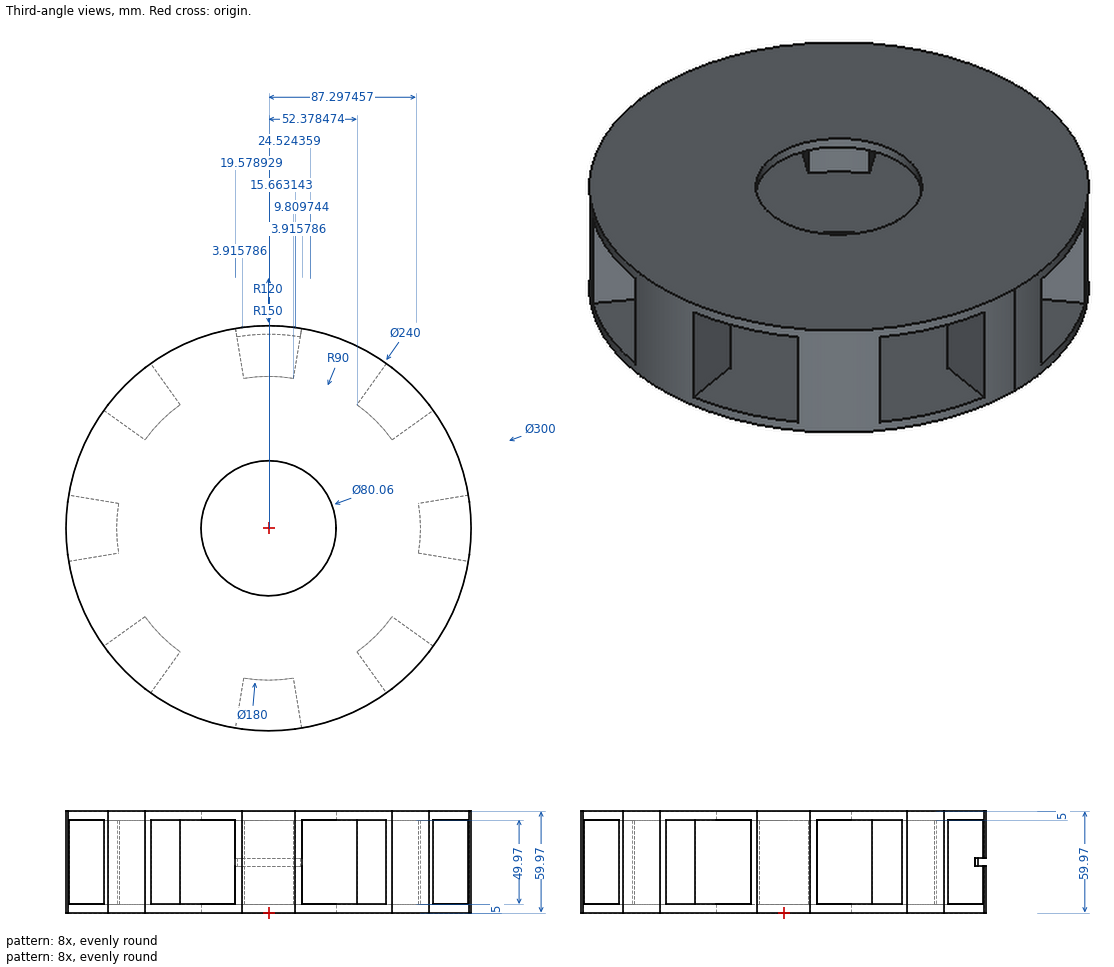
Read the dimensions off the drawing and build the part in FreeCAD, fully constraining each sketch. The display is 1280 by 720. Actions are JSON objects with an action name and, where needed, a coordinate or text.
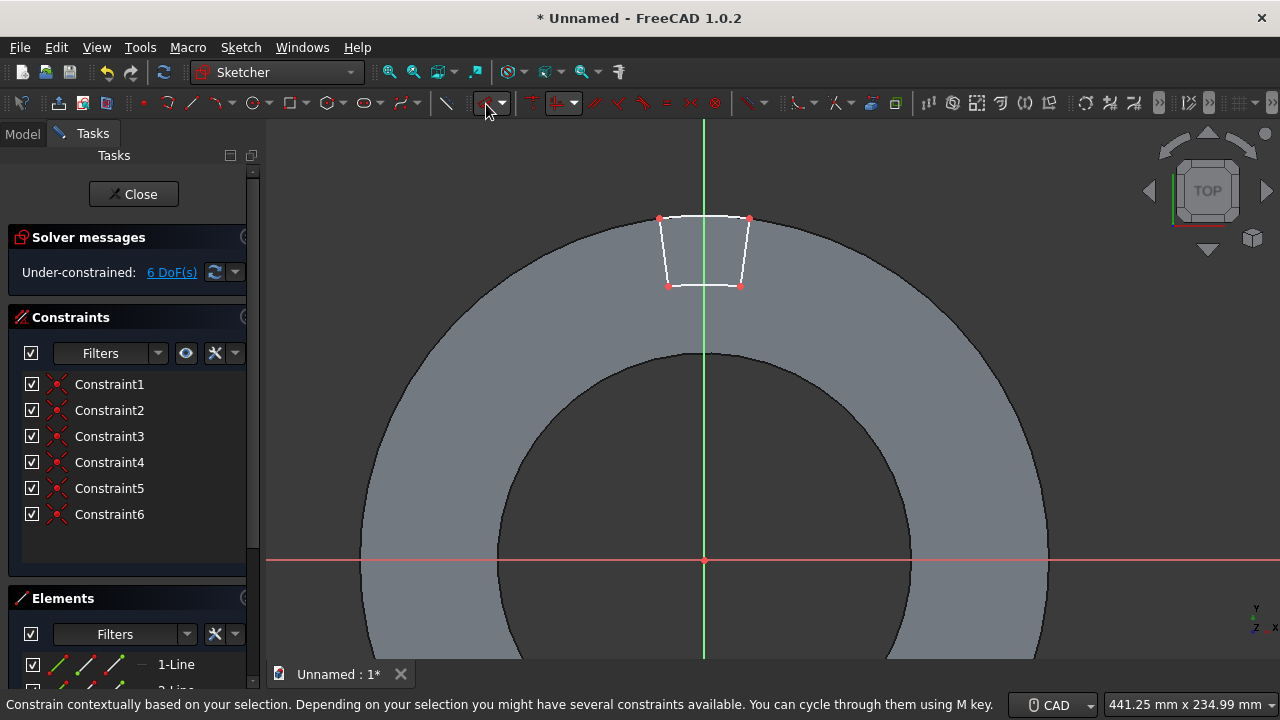
{"action": "left_click", "coordinate": [719, 285]}
{"action": "left_click", "coordinate": [721, 253]}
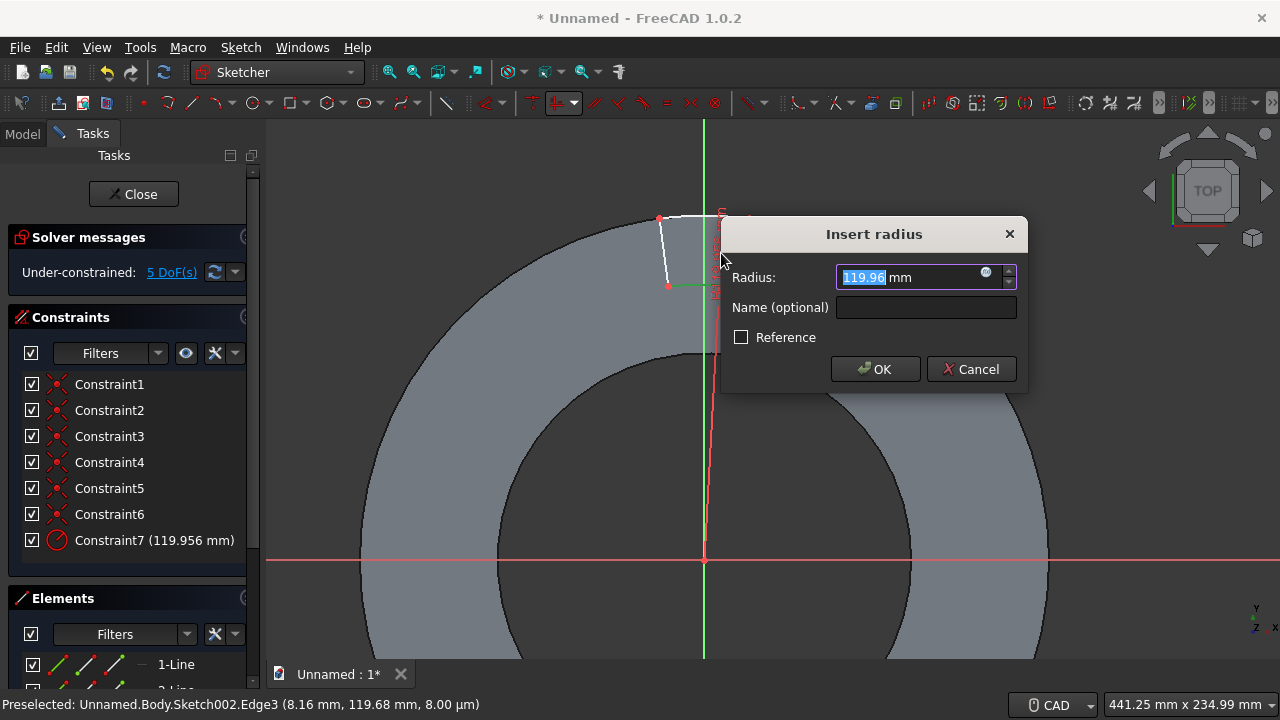
{"action": "type", "text": "120"}
{"action": "key", "text": "Return"}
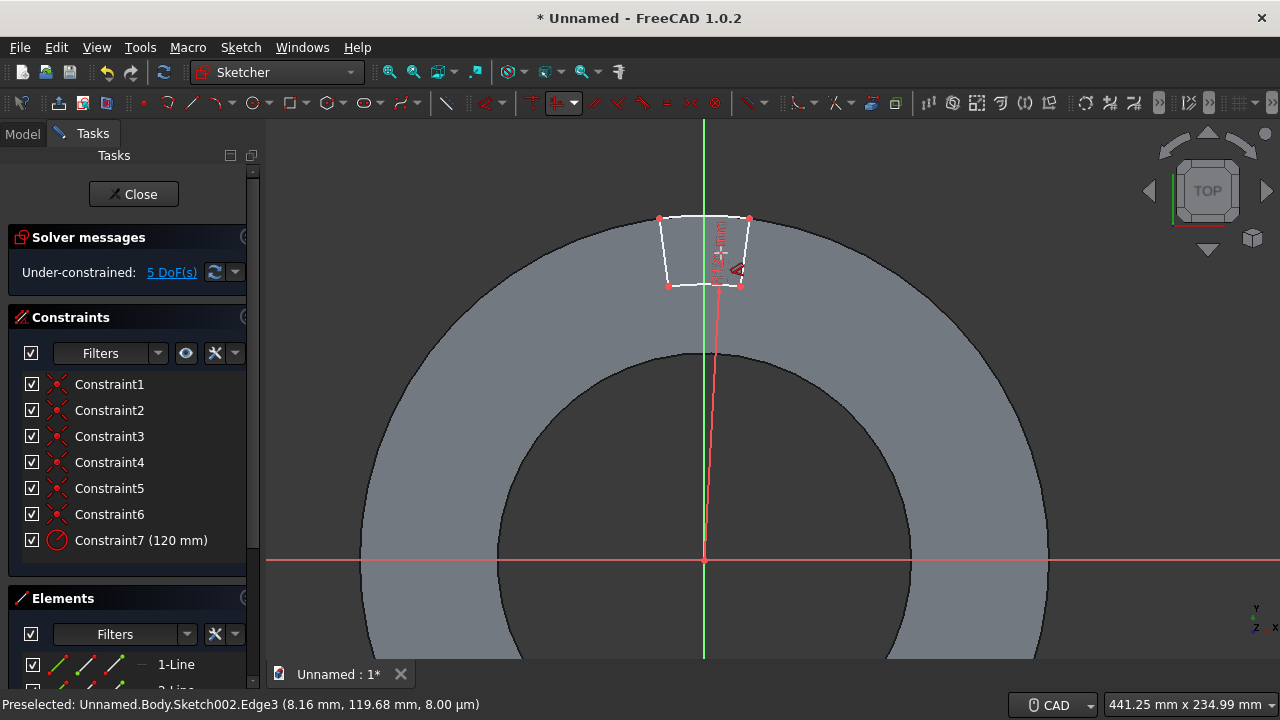
{"action": "left_click", "coordinate": [723, 216]}
{"action": "left_click", "coordinate": [725, 184]}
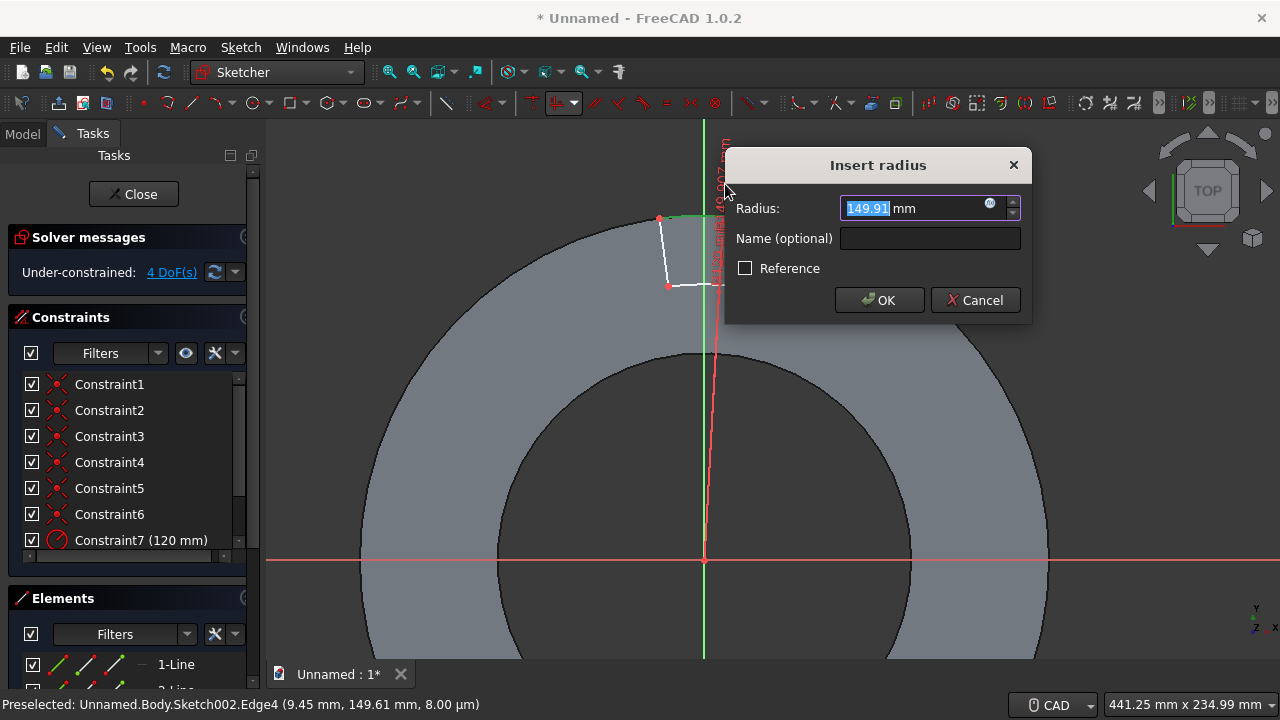
{"action": "type", "text": "150"}
{"action": "key", "text": "Return"}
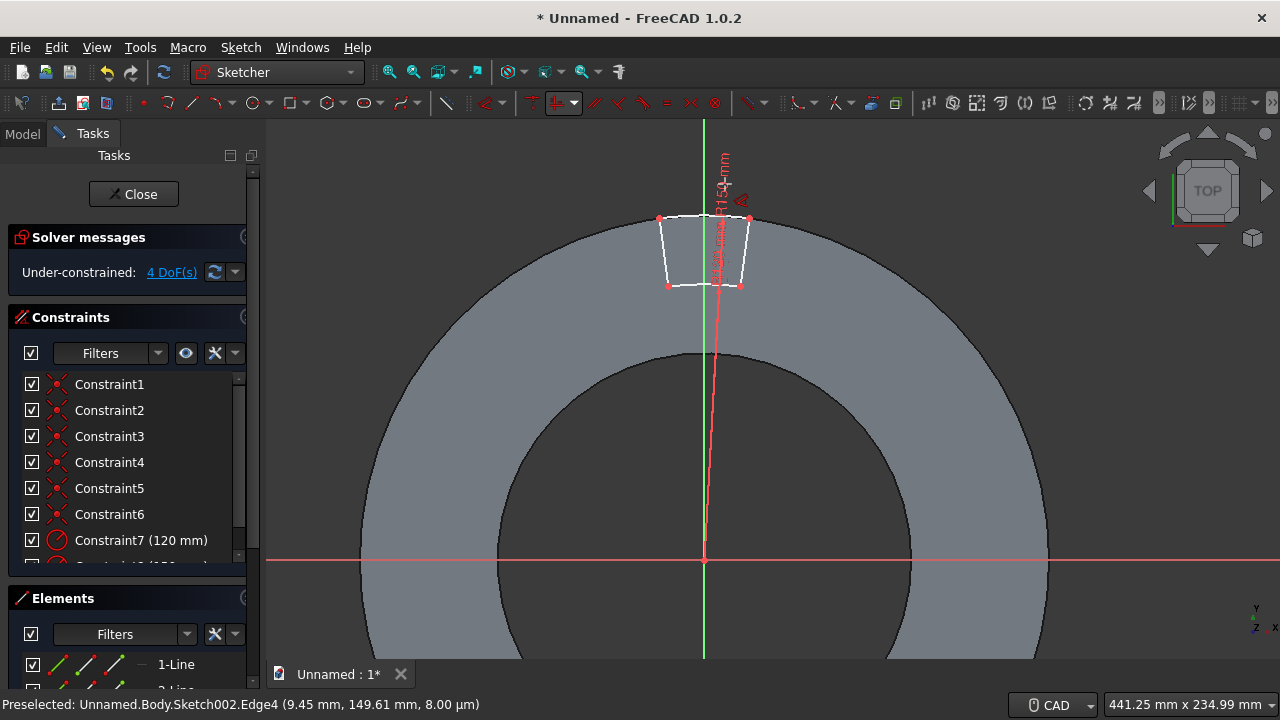
{"action": "scroll", "coordinate": [662, 239], "scroll_direction": "up", "scroll_amount": 8}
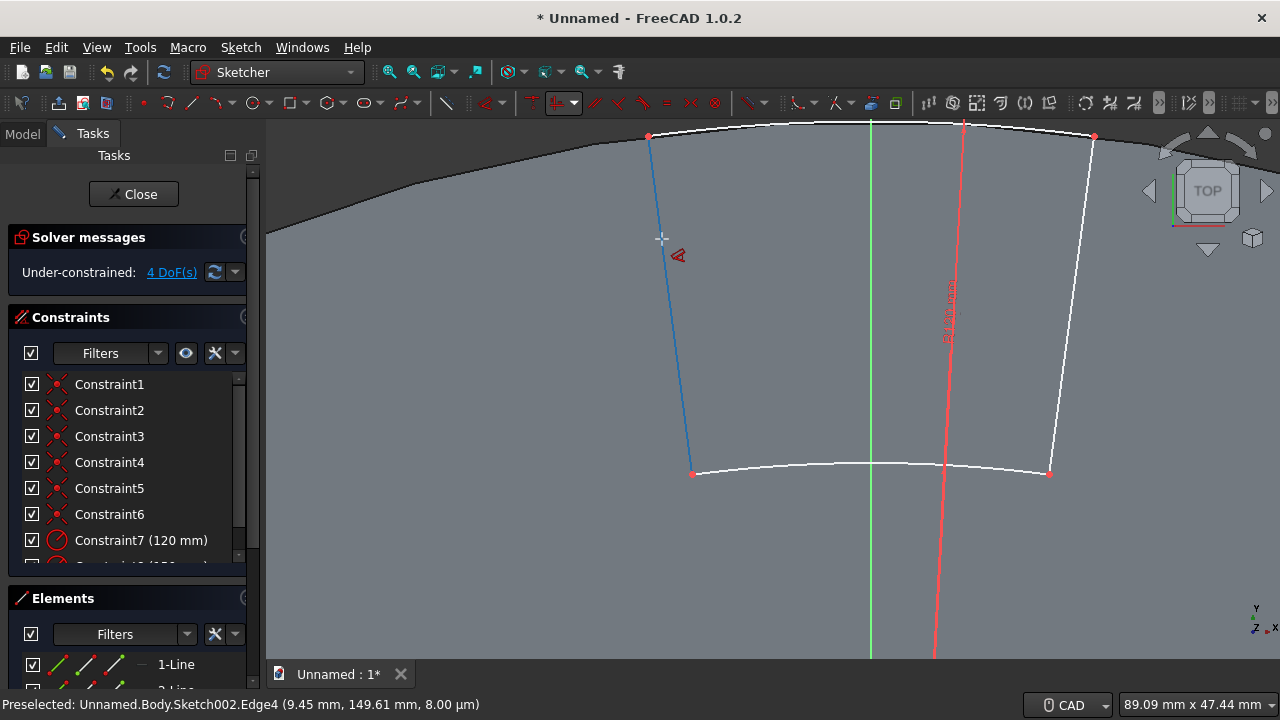
{"action": "left_click", "coordinate": [661, 238]}
{"action": "left_click", "coordinate": [670, 509]}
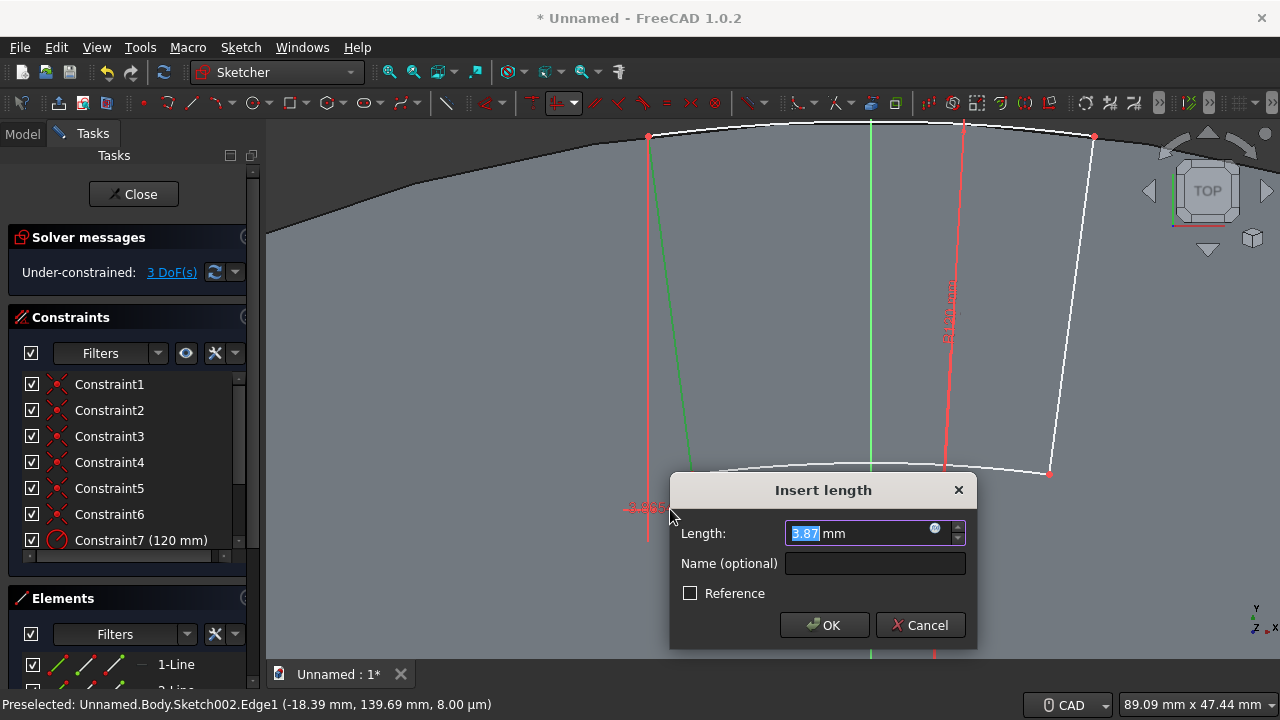
{"action": "type", "text": "3.915786"}
{"action": "key", "text": "Return"}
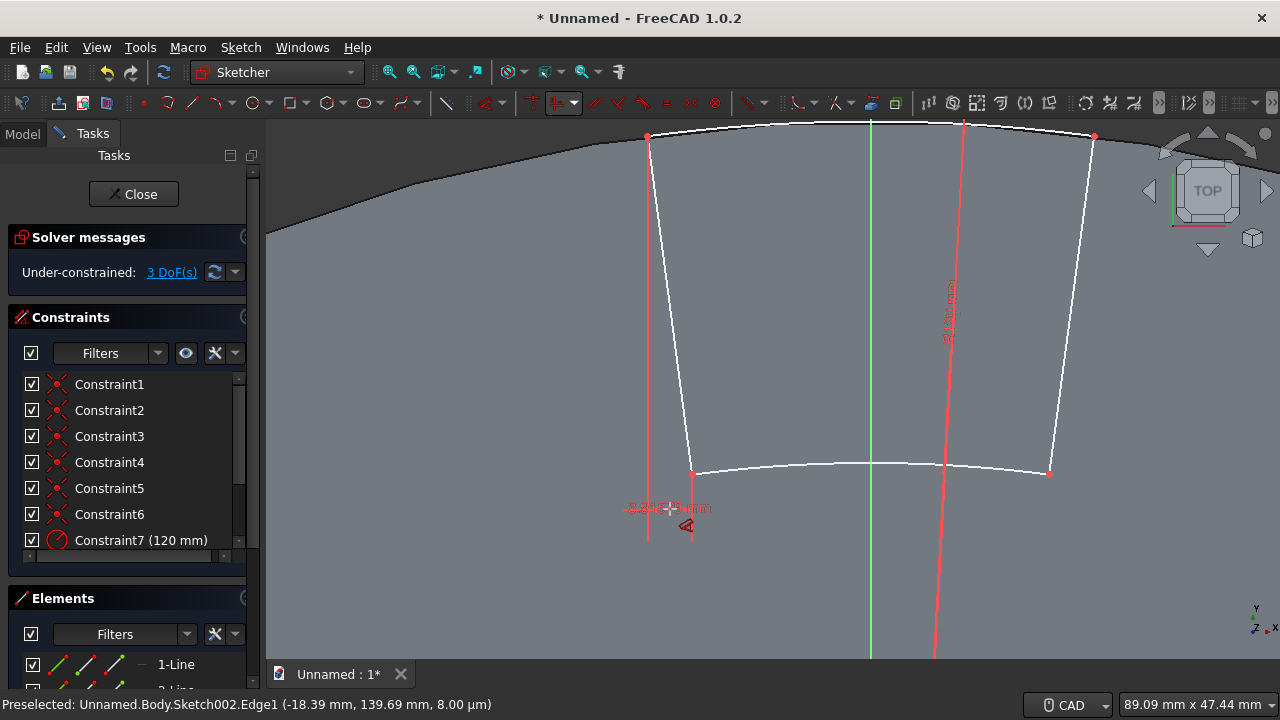
{"action": "left_click", "coordinate": [1063, 373]}
{"action": "left_click", "coordinate": [1072, 509]}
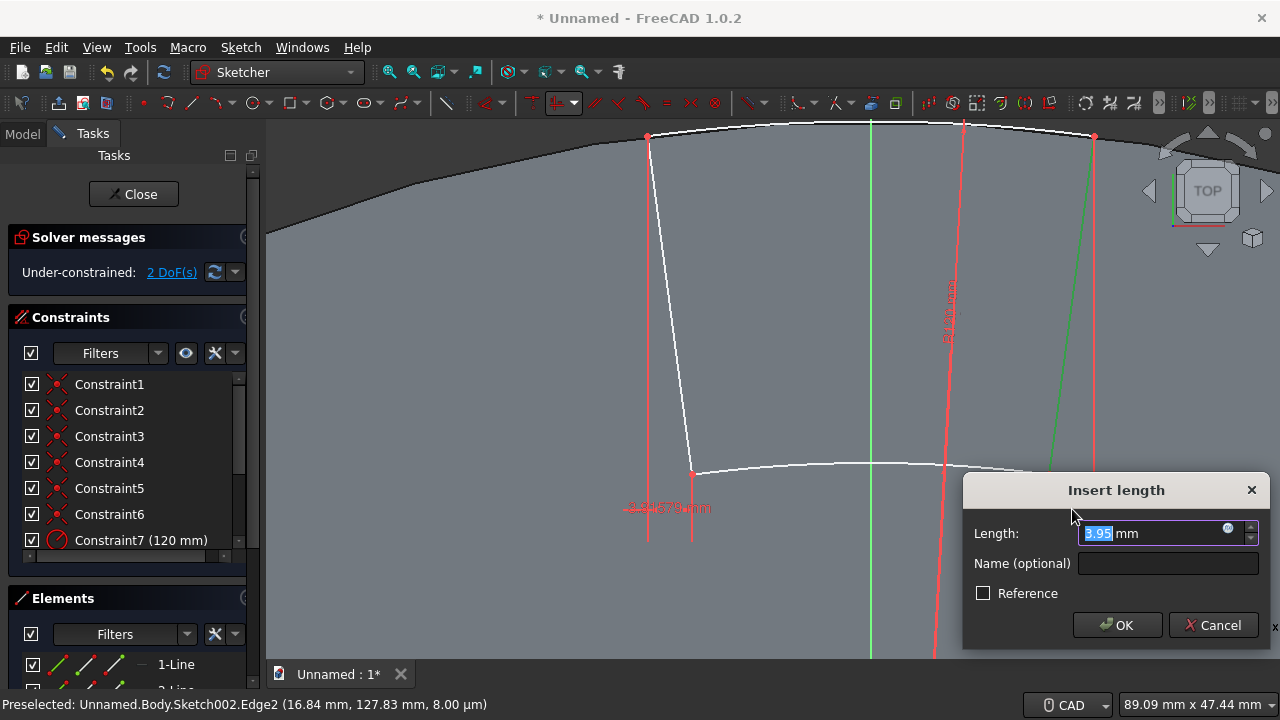
{"action": "type", "text": "3.915786"}
{"action": "key", "text": "Return"}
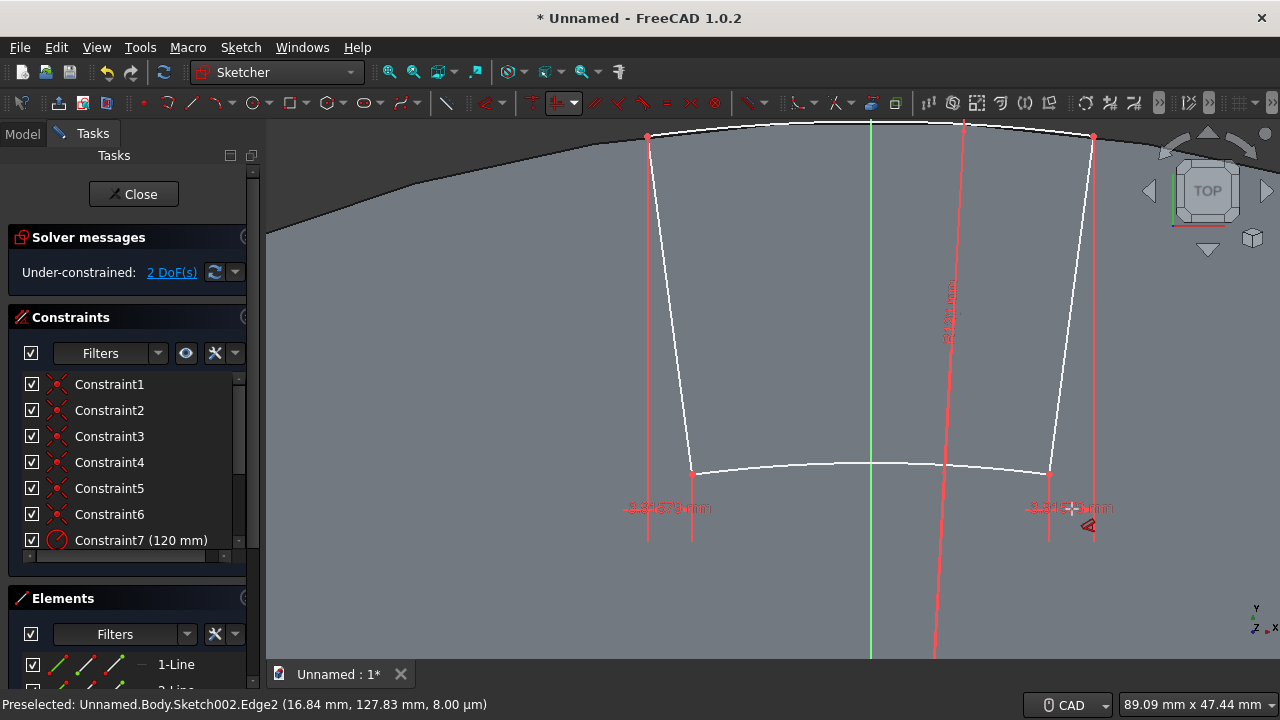
{"action": "scroll", "coordinate": [294, 631], "scroll_direction": "down", "scroll_amount": 1}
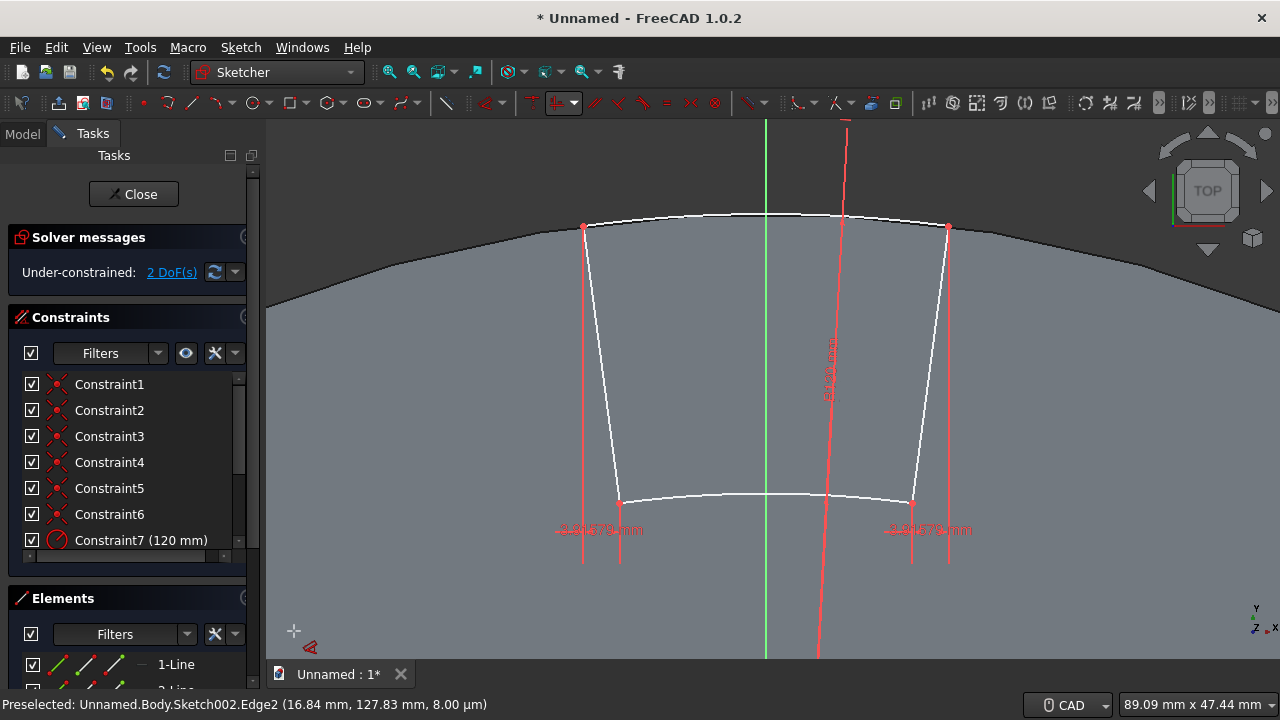
{"action": "left_click", "coordinate": [583, 226]}
{"action": "left_click", "coordinate": [675, 192]}